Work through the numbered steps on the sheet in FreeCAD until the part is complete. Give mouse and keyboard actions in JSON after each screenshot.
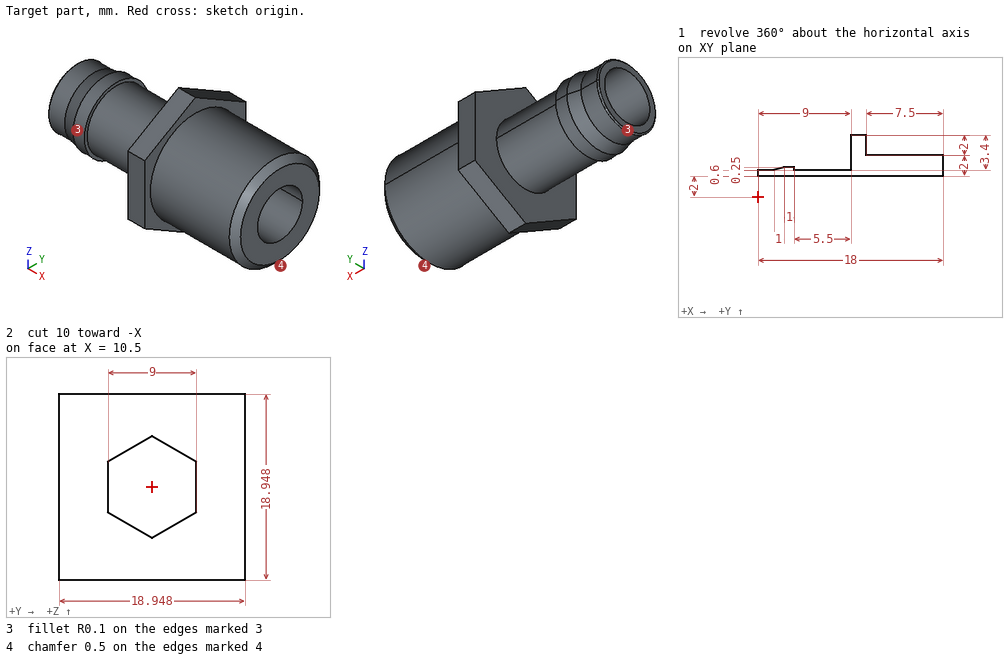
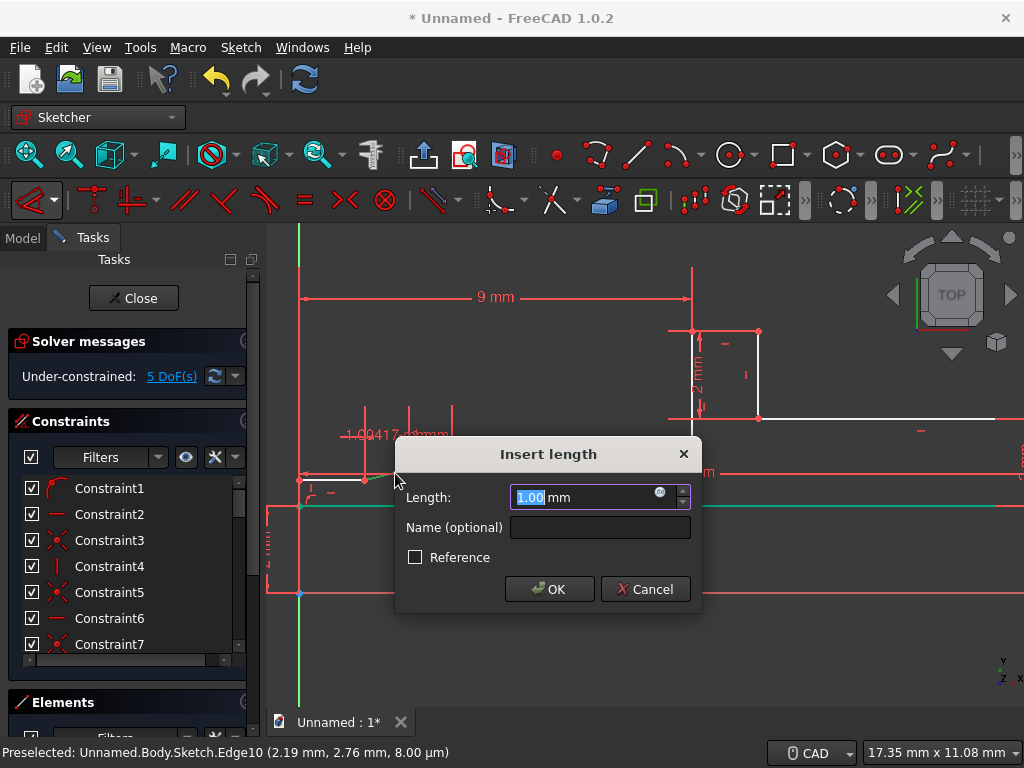
{"action": "type", "text": "1"}
{"action": "key", "text": "Return"}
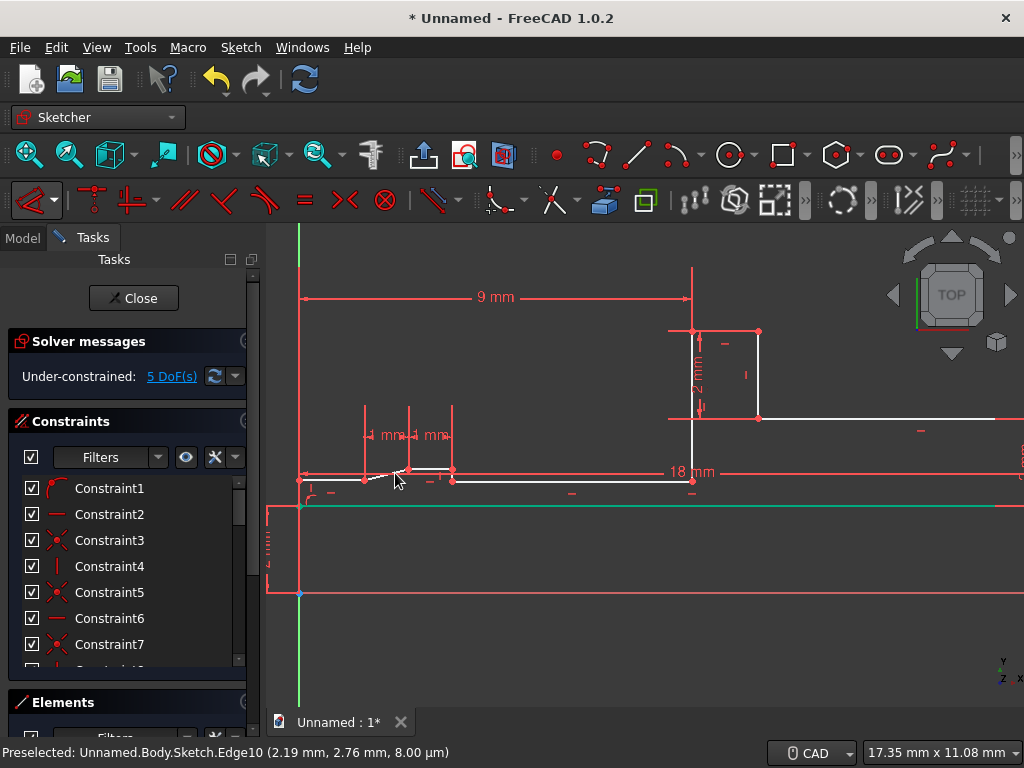
{"action": "left_click", "coordinate": [856, 419]}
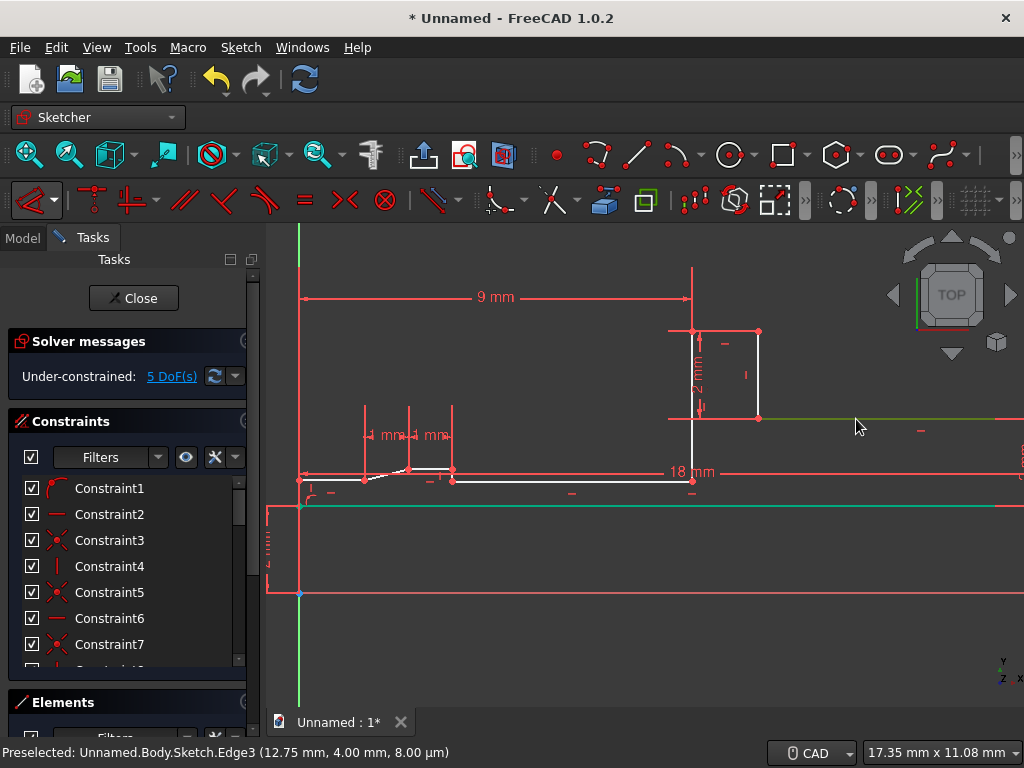
{"action": "left_click", "coordinate": [56, 200]}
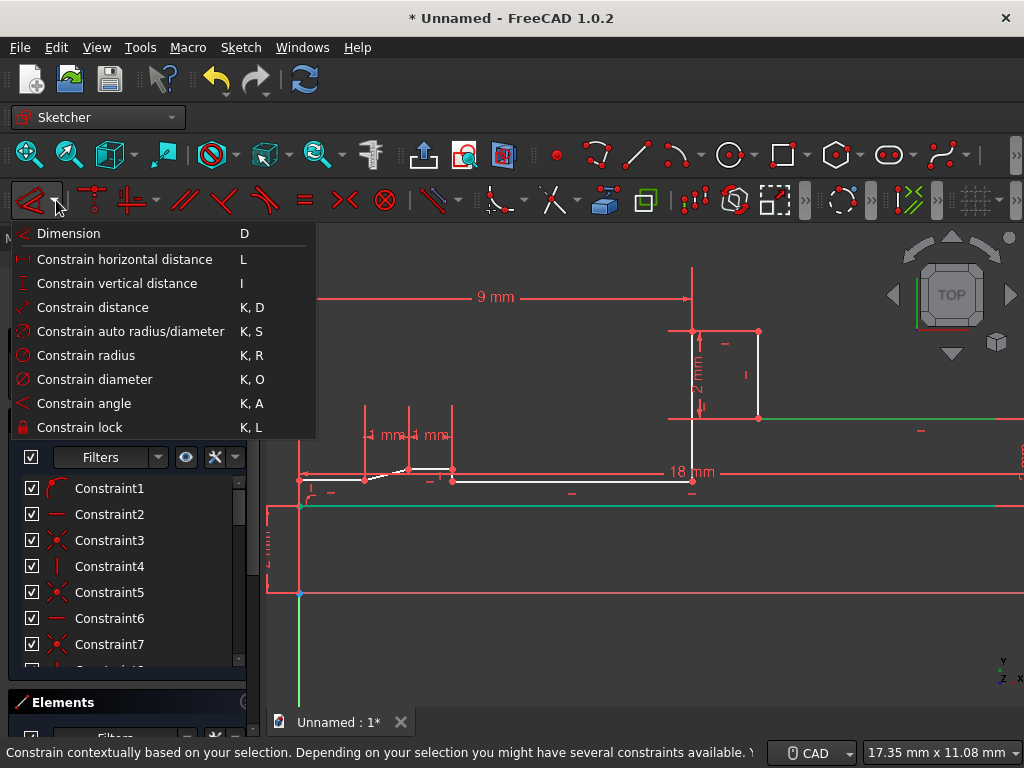
{"action": "left_click", "coordinate": [164, 259]}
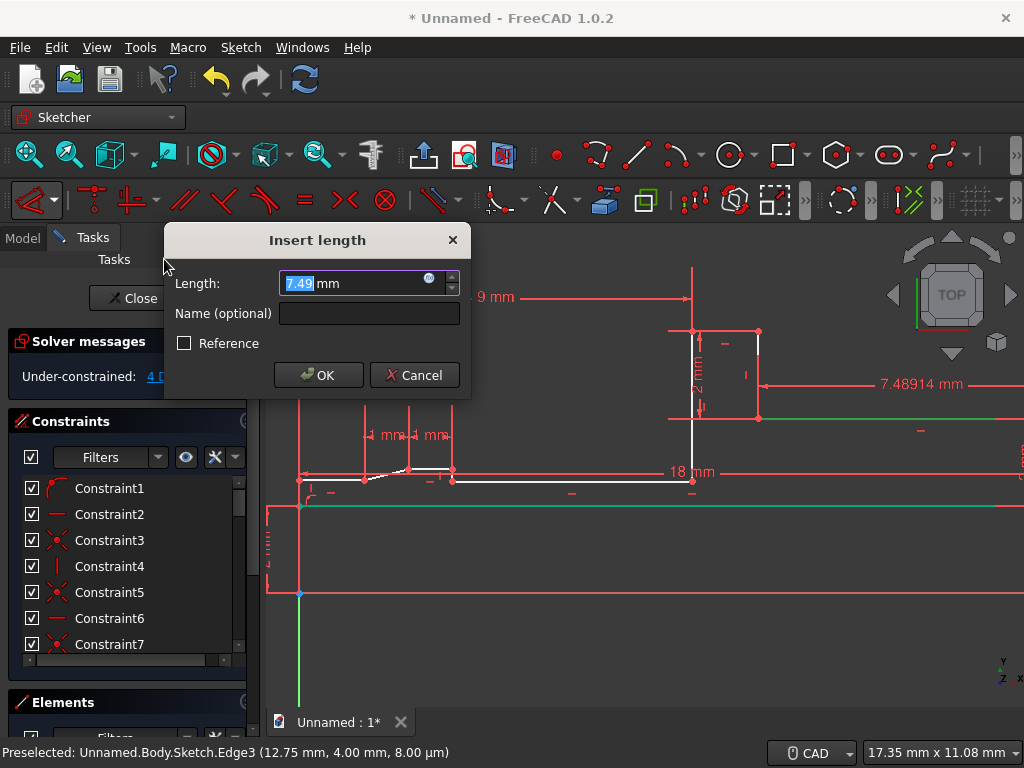
{"action": "type", "text": "7.5"}
{"action": "key", "text": "Return"}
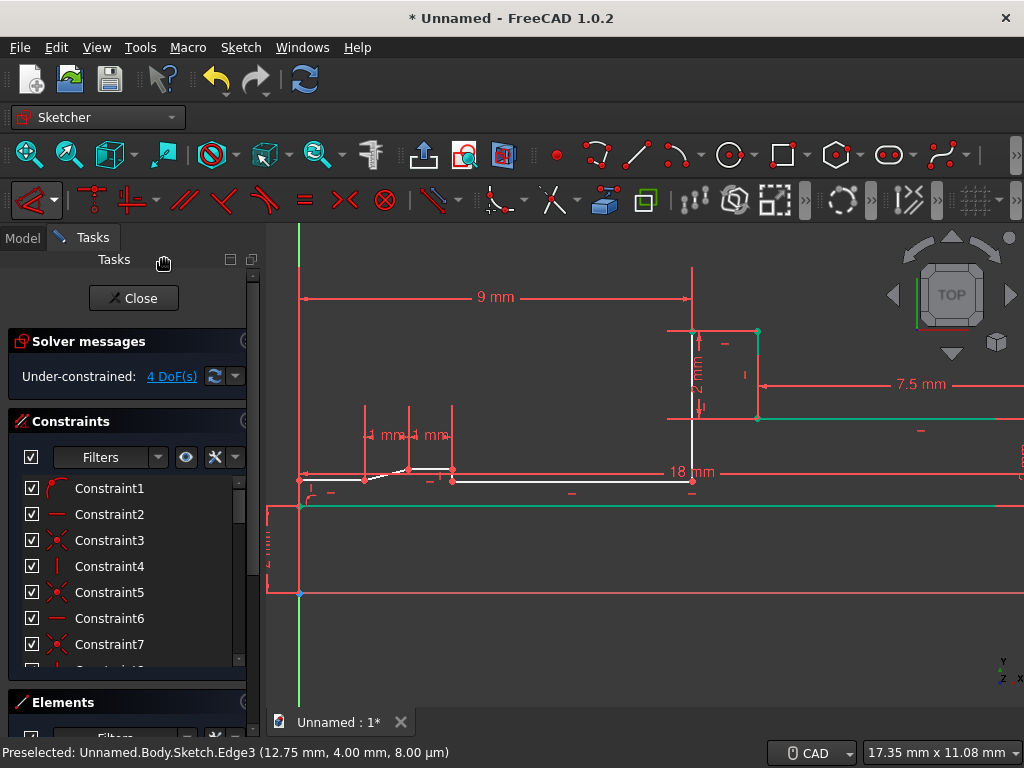
{"action": "left_click", "coordinate": [692, 437]}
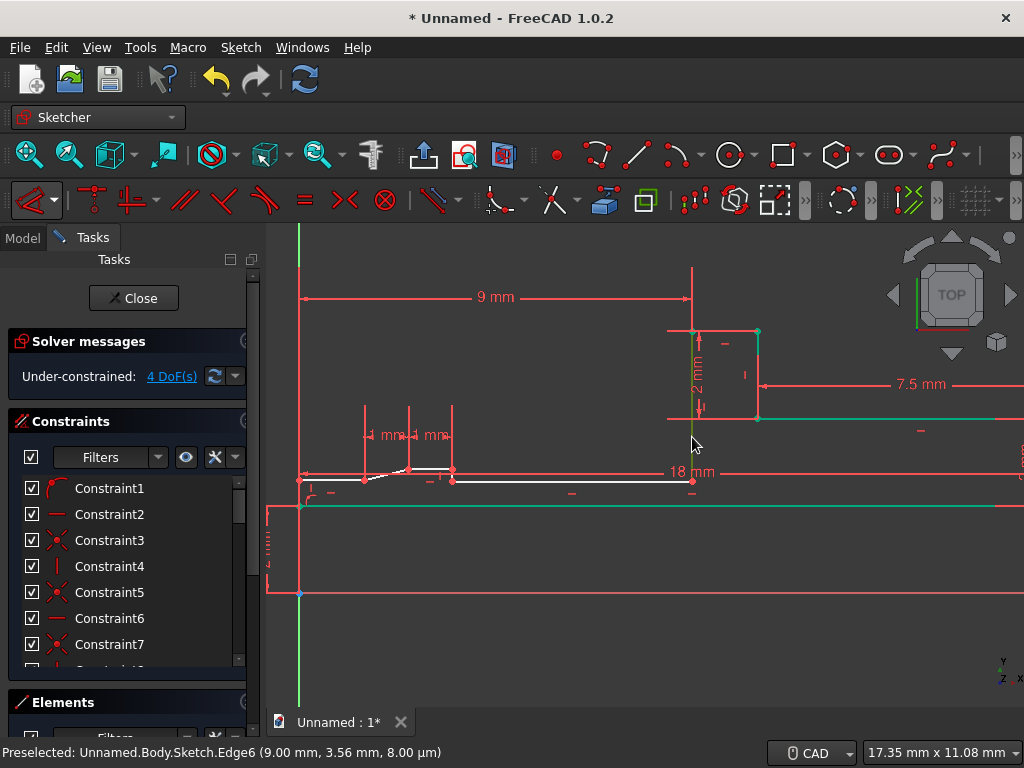
{"action": "left_click", "coordinate": [56, 200]}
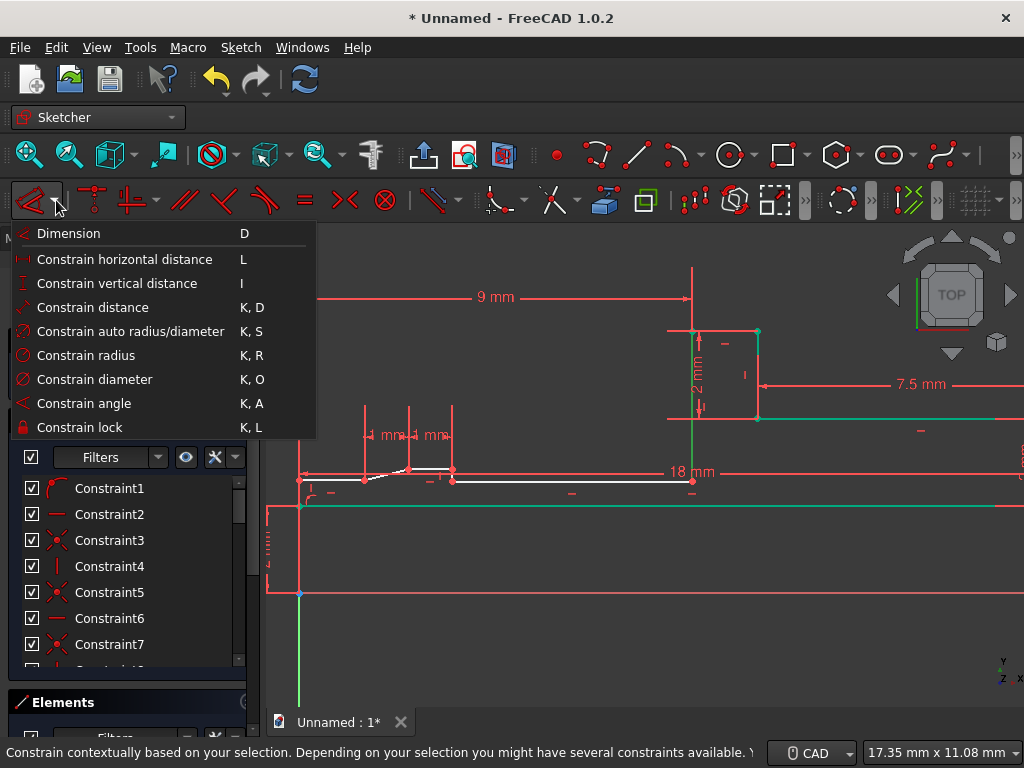
{"action": "left_click", "coordinate": [164, 283]}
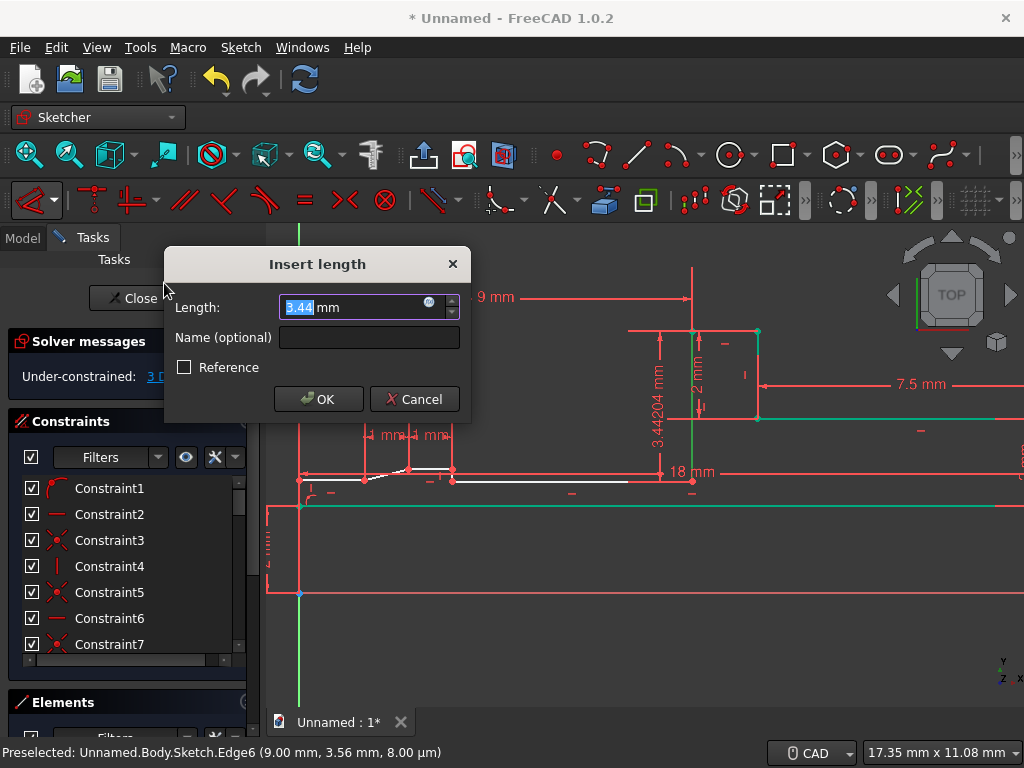
{"action": "type", "text": "3.4"}
{"action": "key", "text": "Return"}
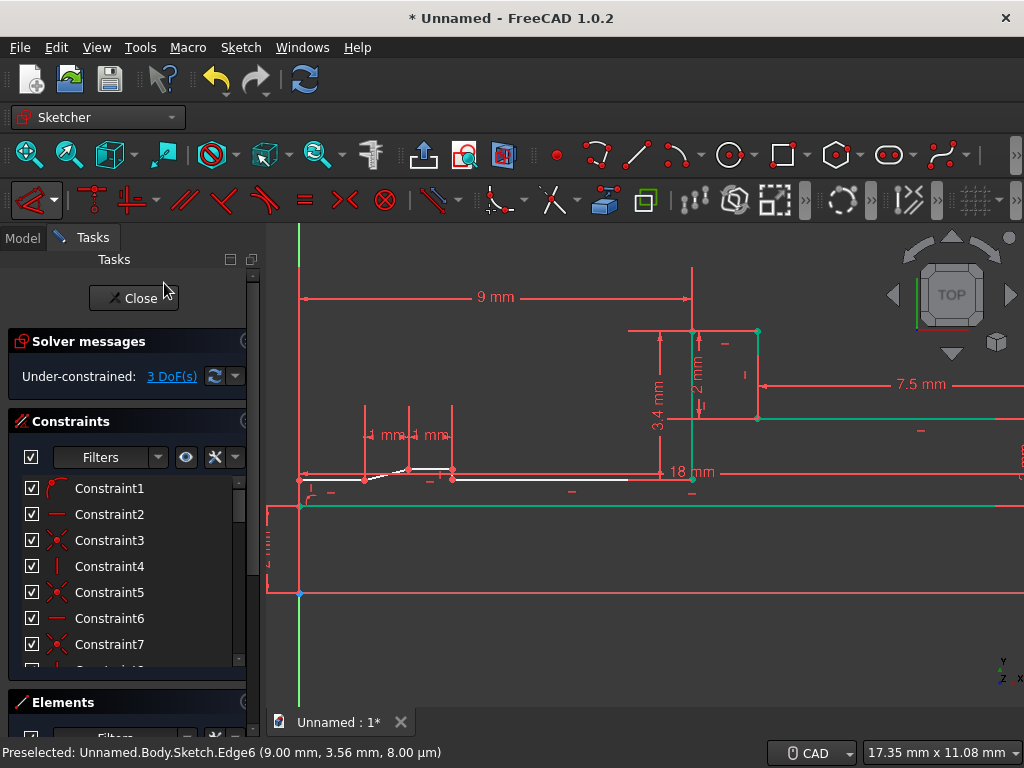
{"action": "left_click", "coordinate": [620, 480]}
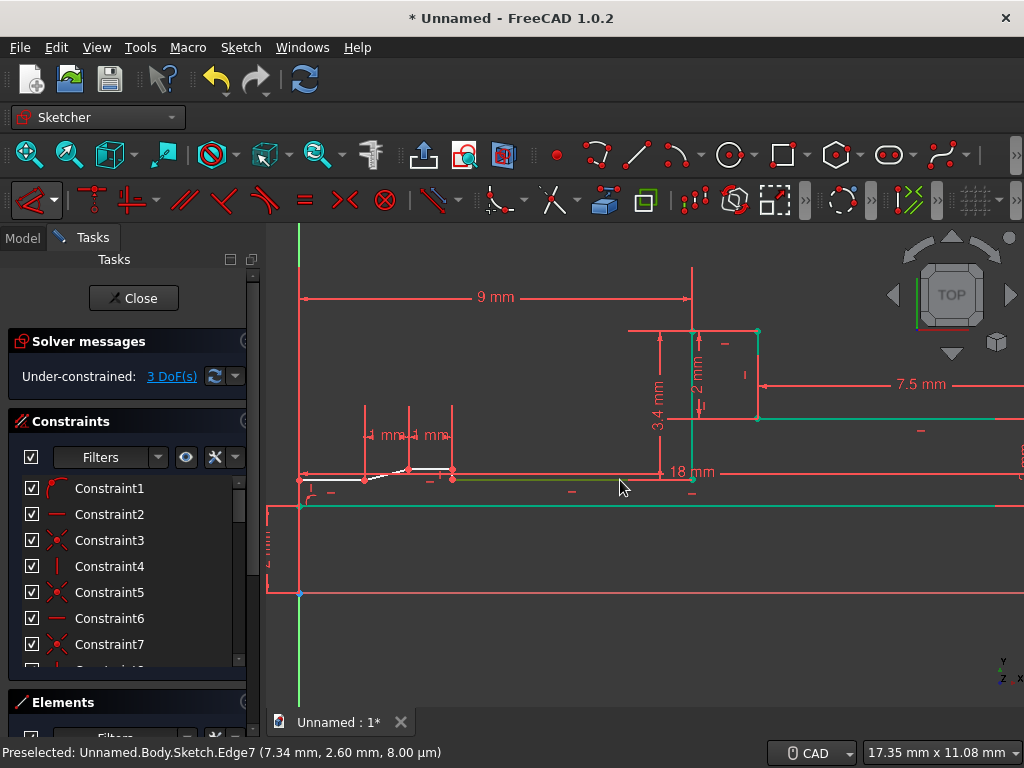
{"action": "key", "text": "l"}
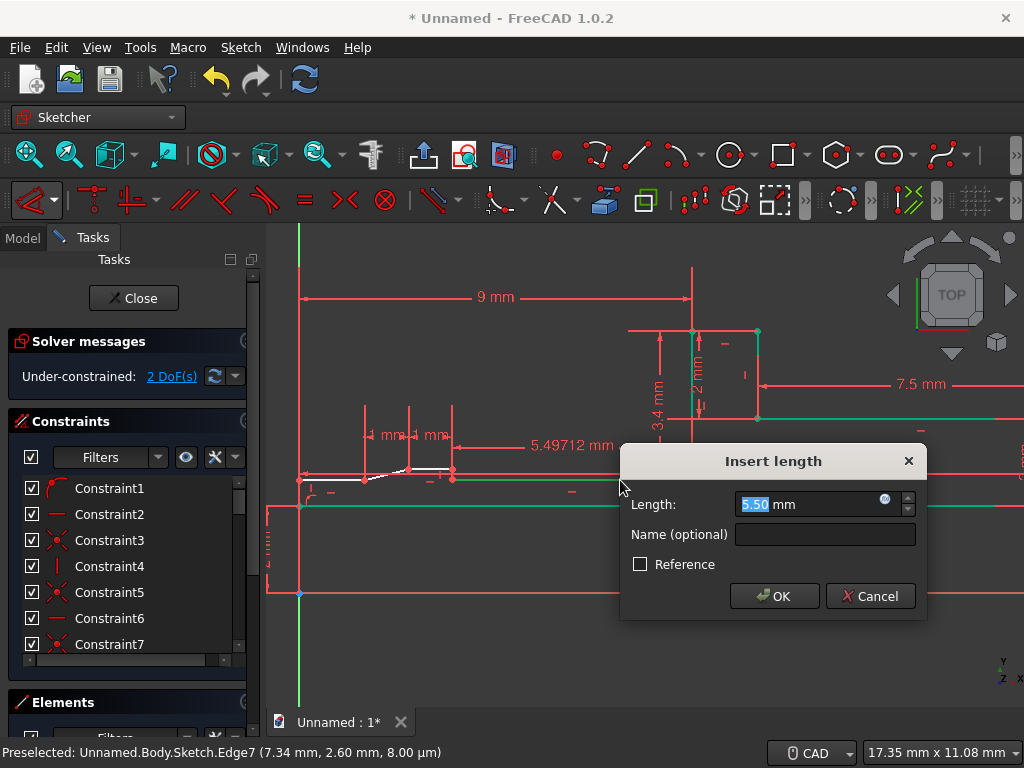
{"action": "type", "text": "5.5"}
{"action": "key", "text": "Return"}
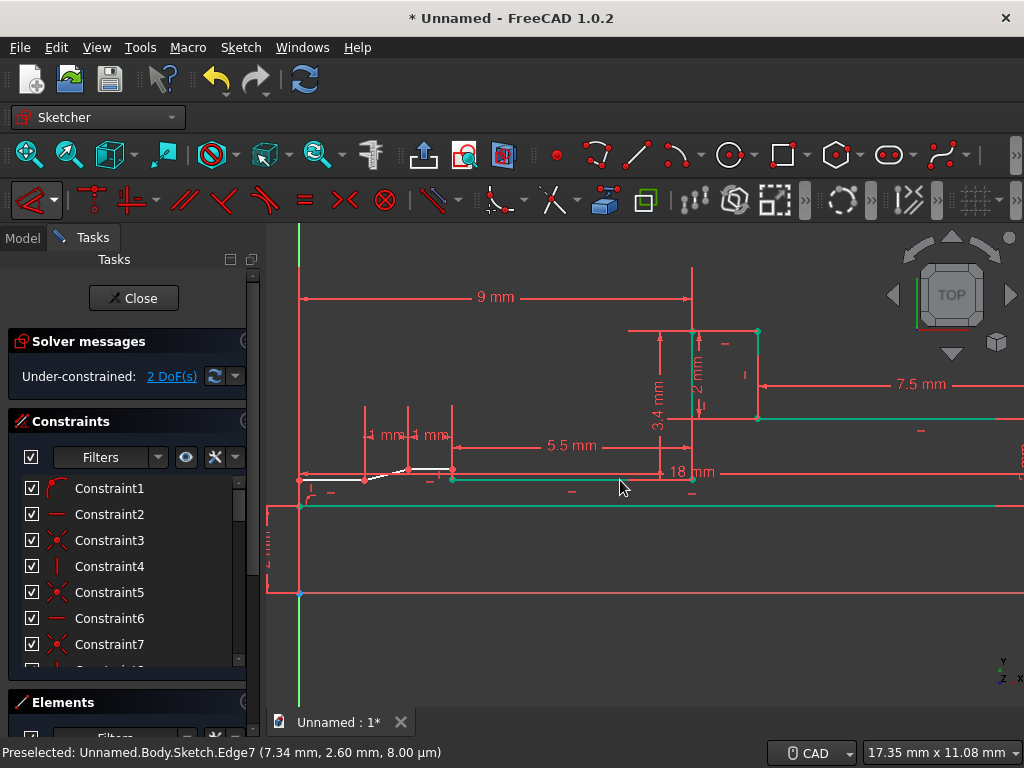
{"action": "scroll", "coordinate": [299, 491], "scroll_direction": "up", "scroll_amount": 3}